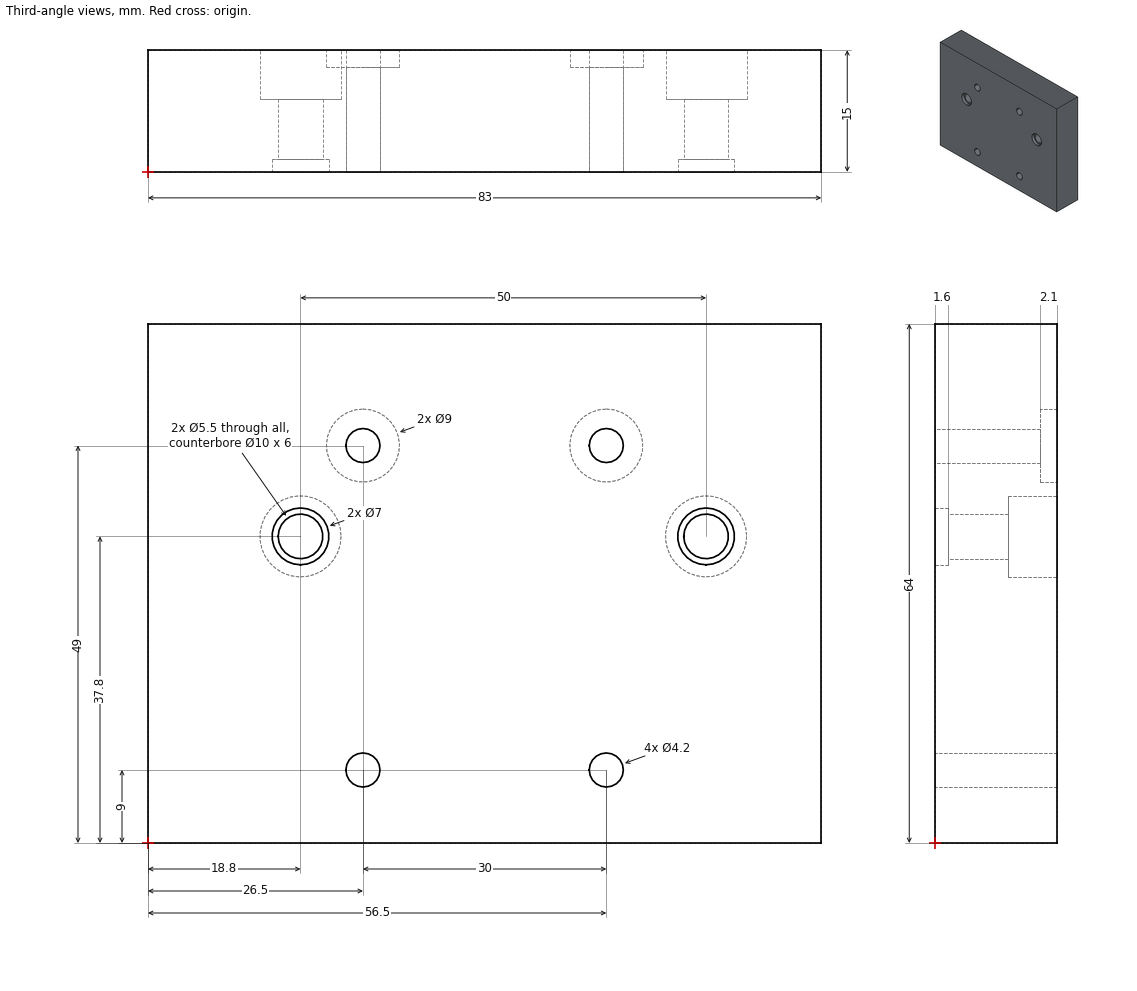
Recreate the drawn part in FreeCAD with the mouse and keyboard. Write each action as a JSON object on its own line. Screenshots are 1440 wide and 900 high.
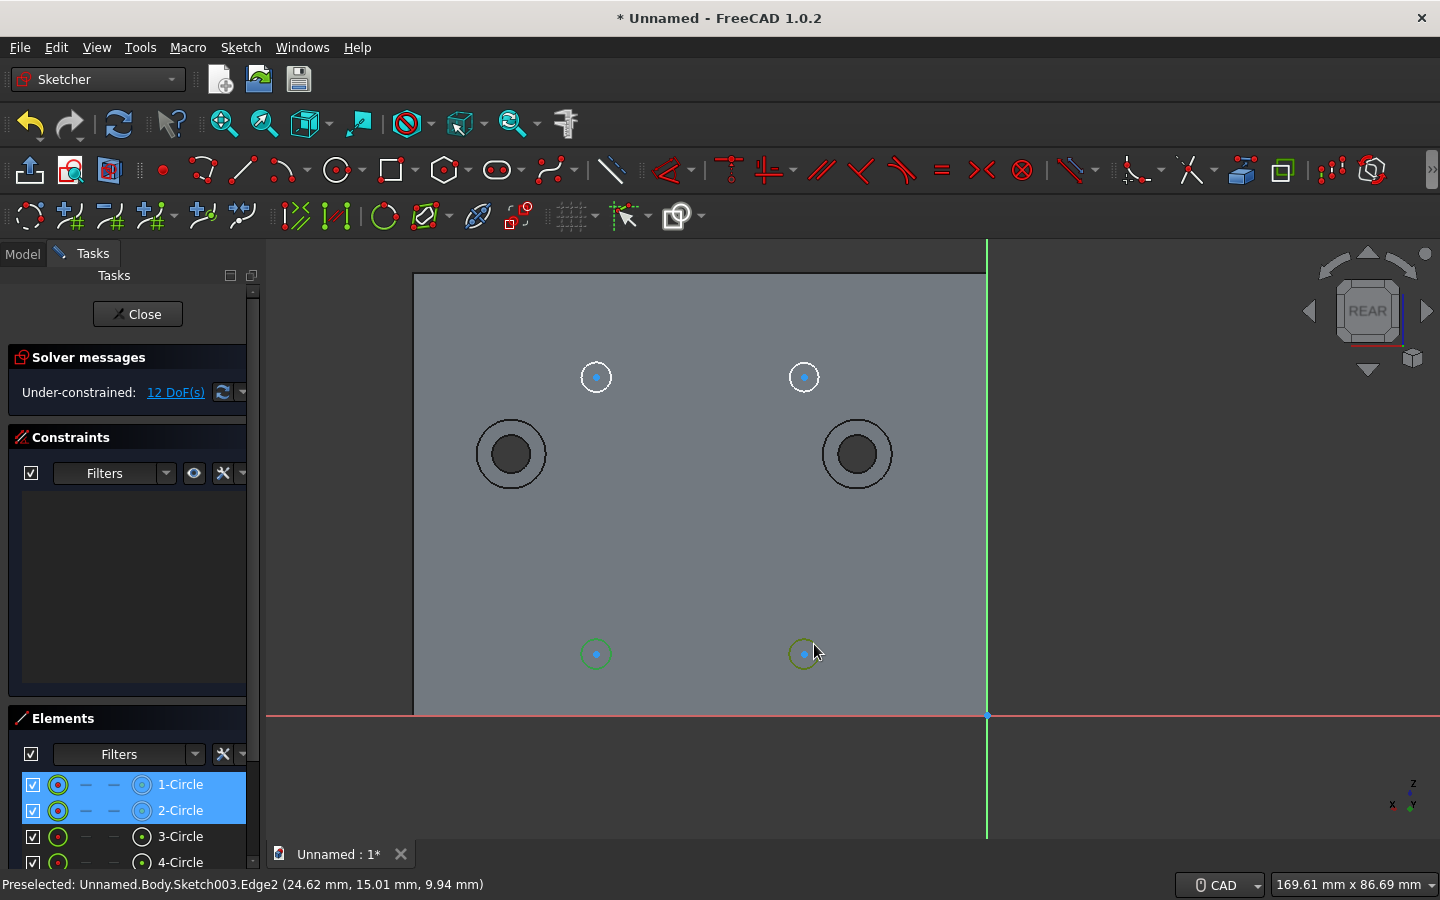
{"action": "left_click", "coordinate": [814, 367]}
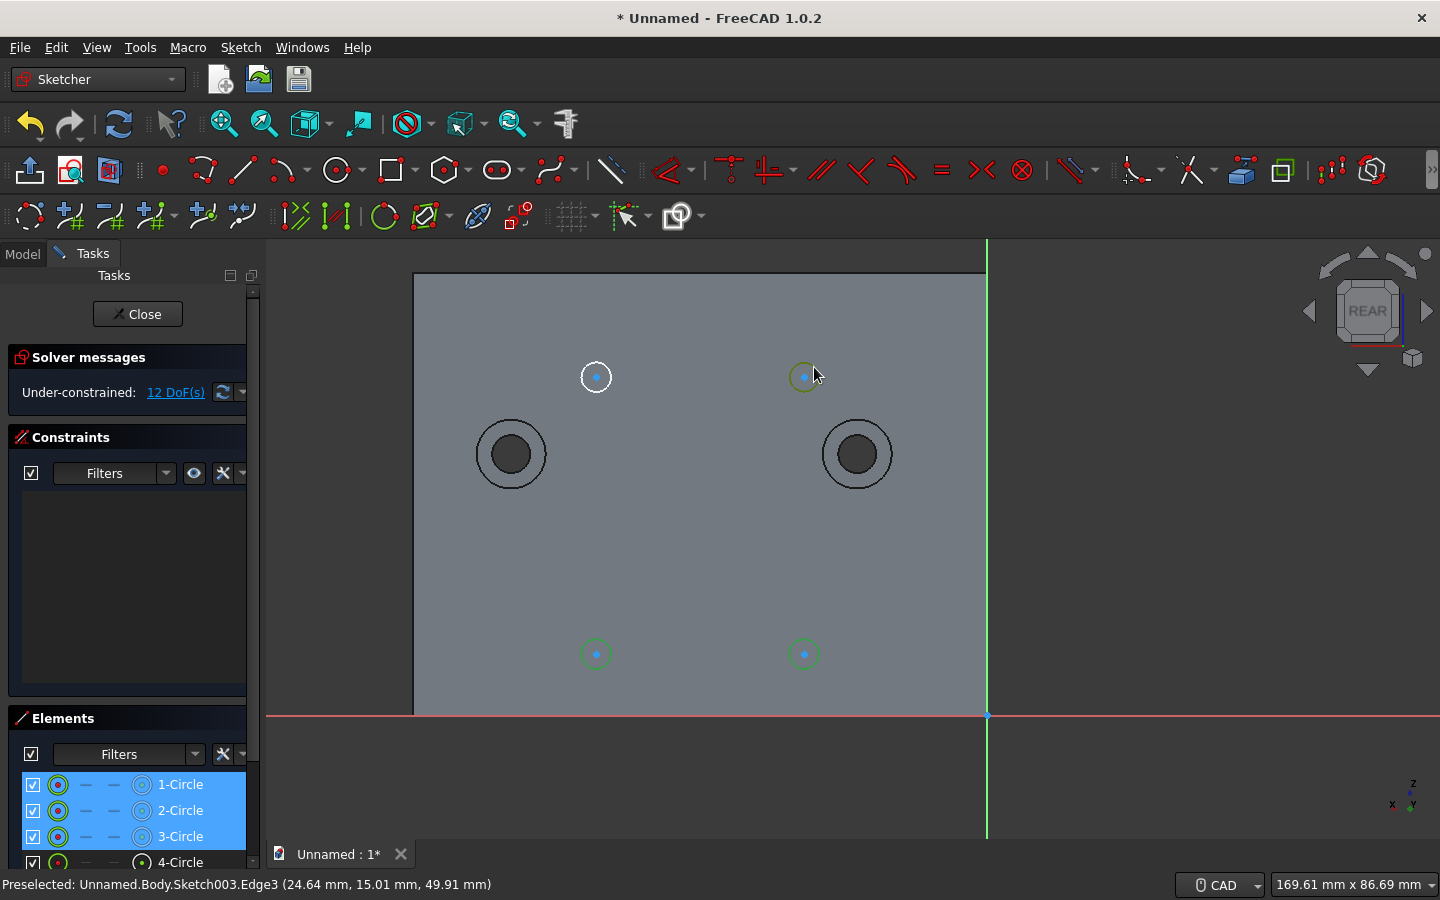
{"action": "left_click", "coordinate": [607, 367]}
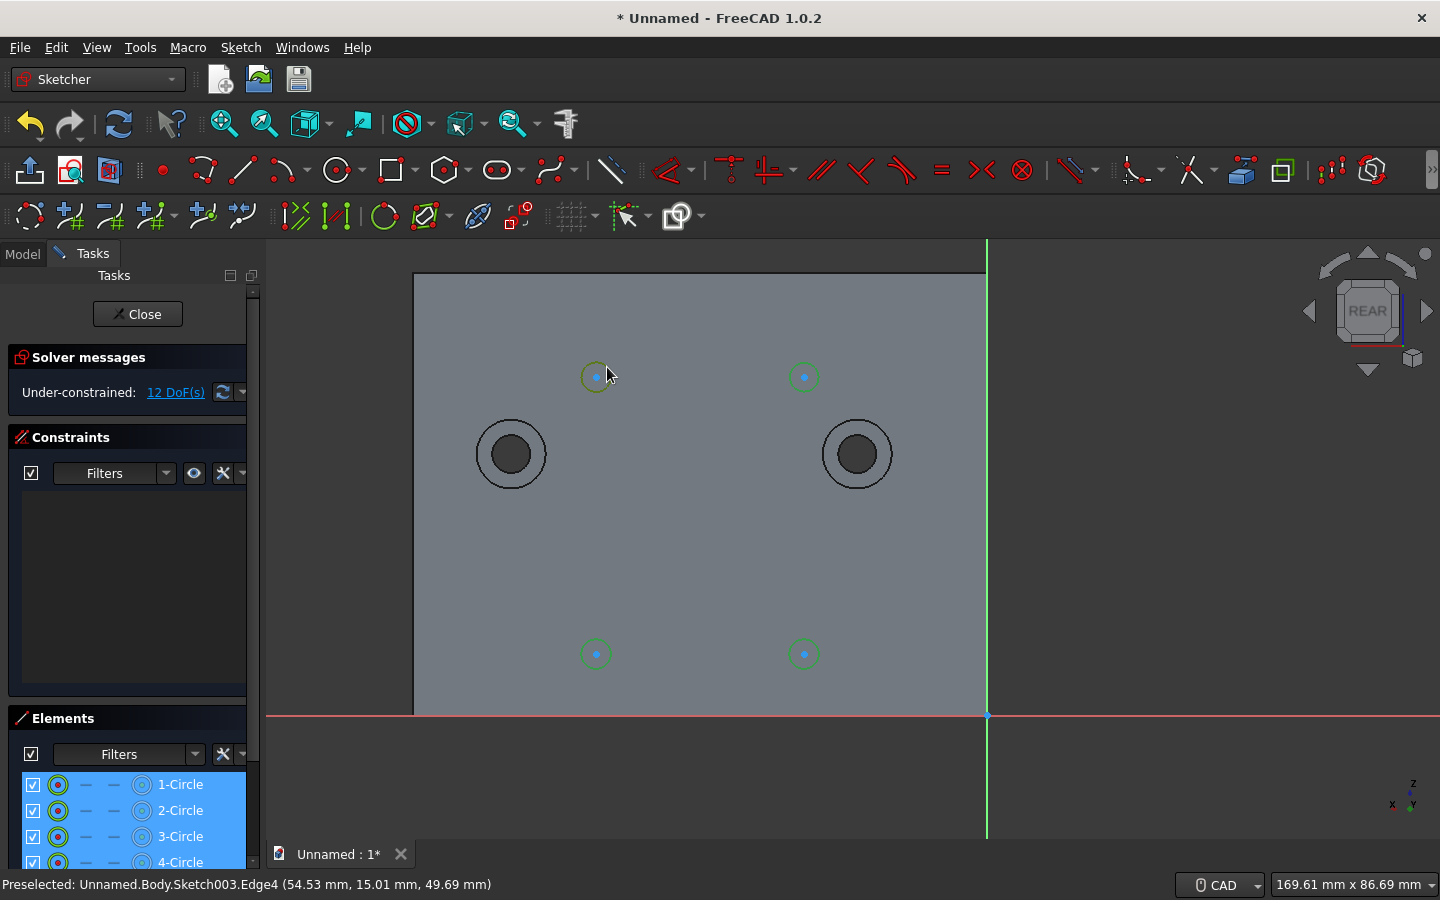
{"action": "left_click", "coordinate": [942, 170]}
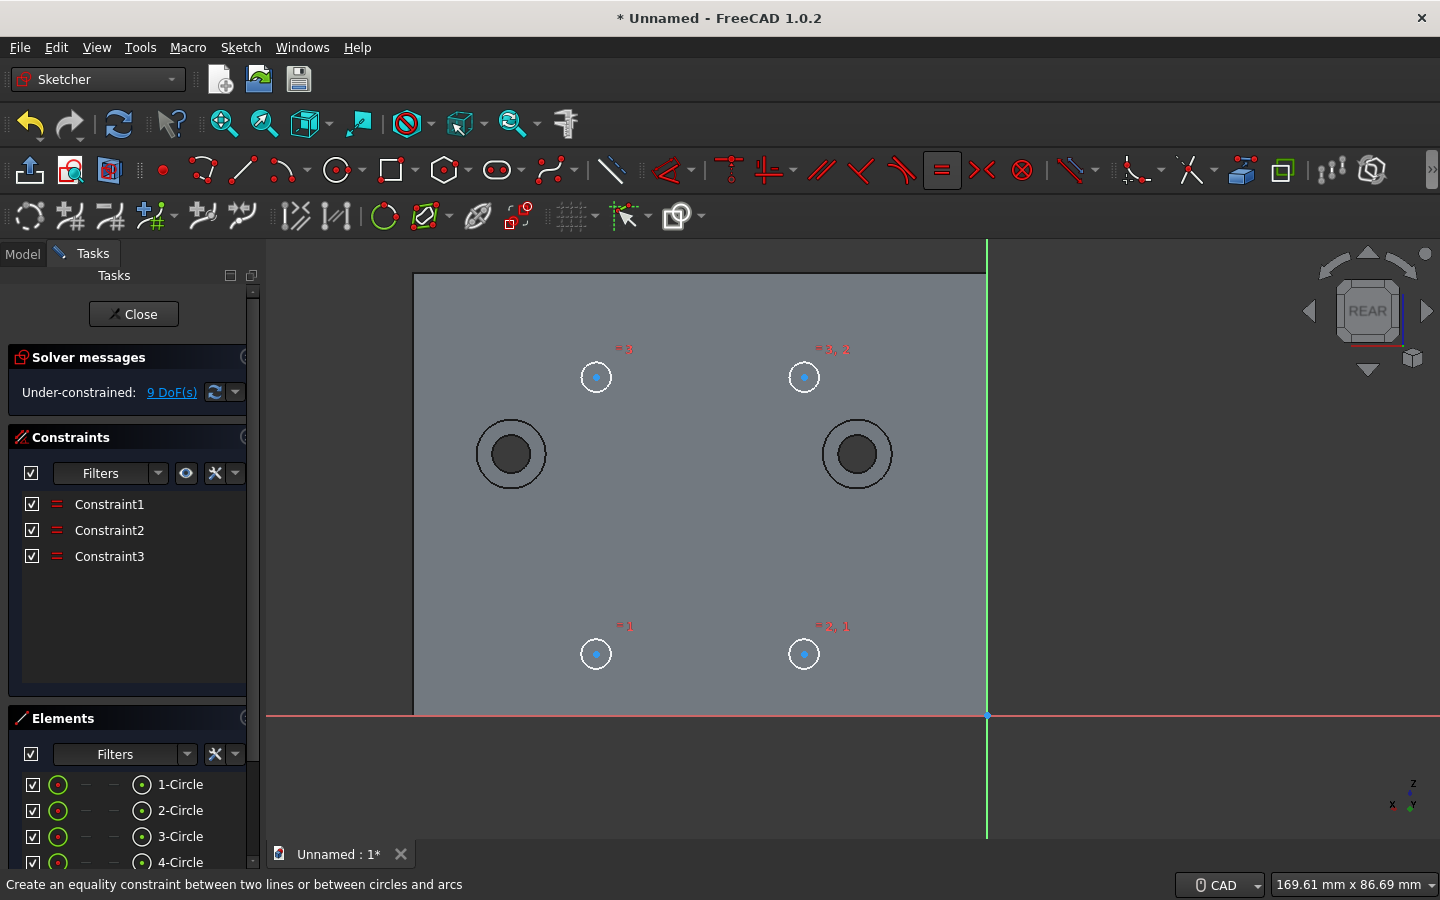
{"action": "left_click", "coordinate": [666, 170]}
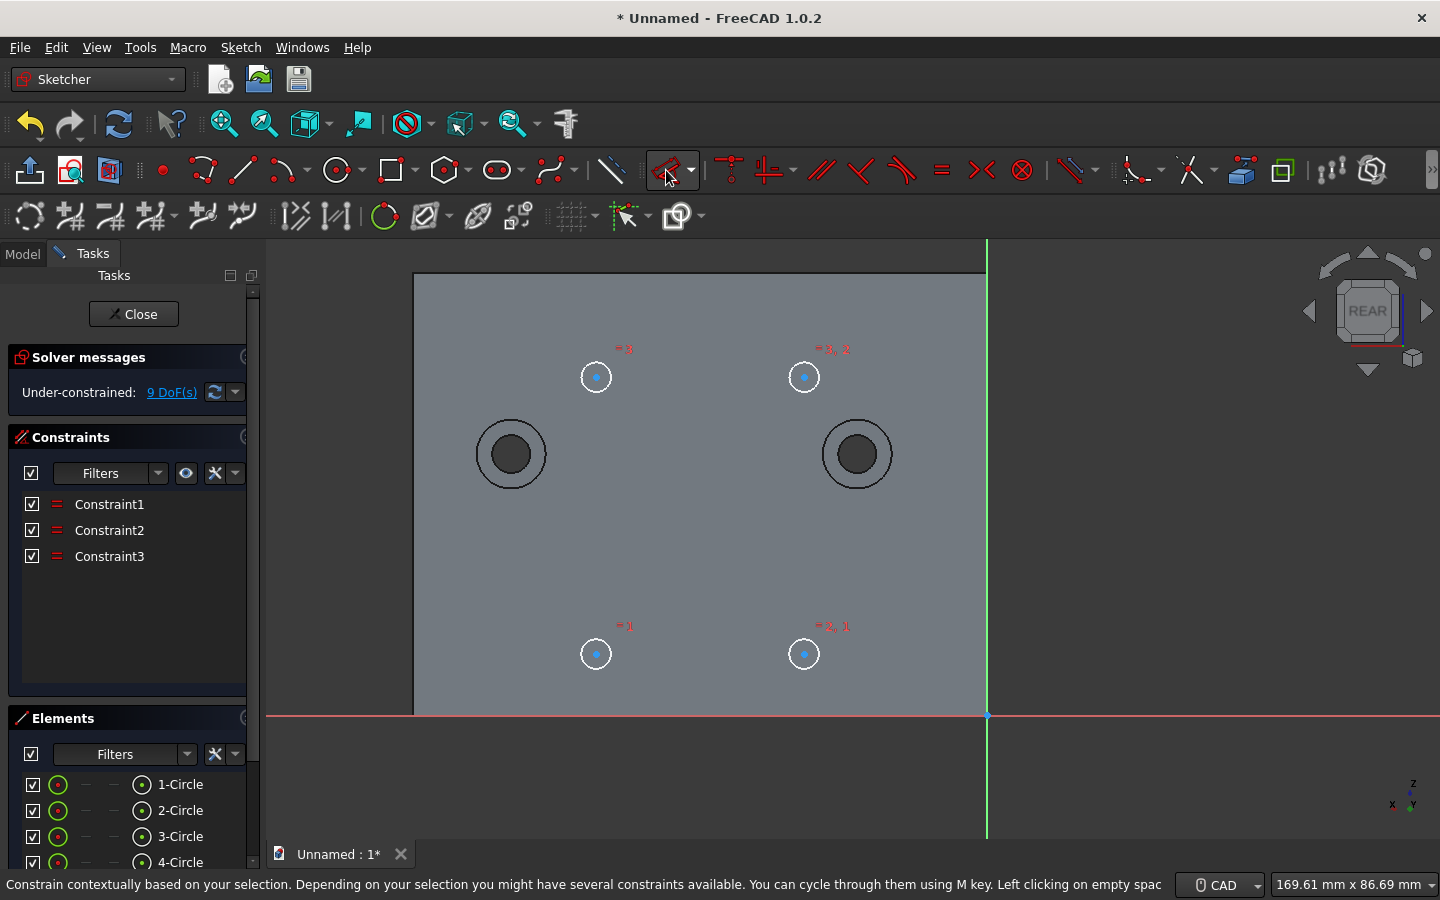
{"action": "scroll", "coordinate": [606, 644], "scroll_direction": "up", "scroll_amount": 2}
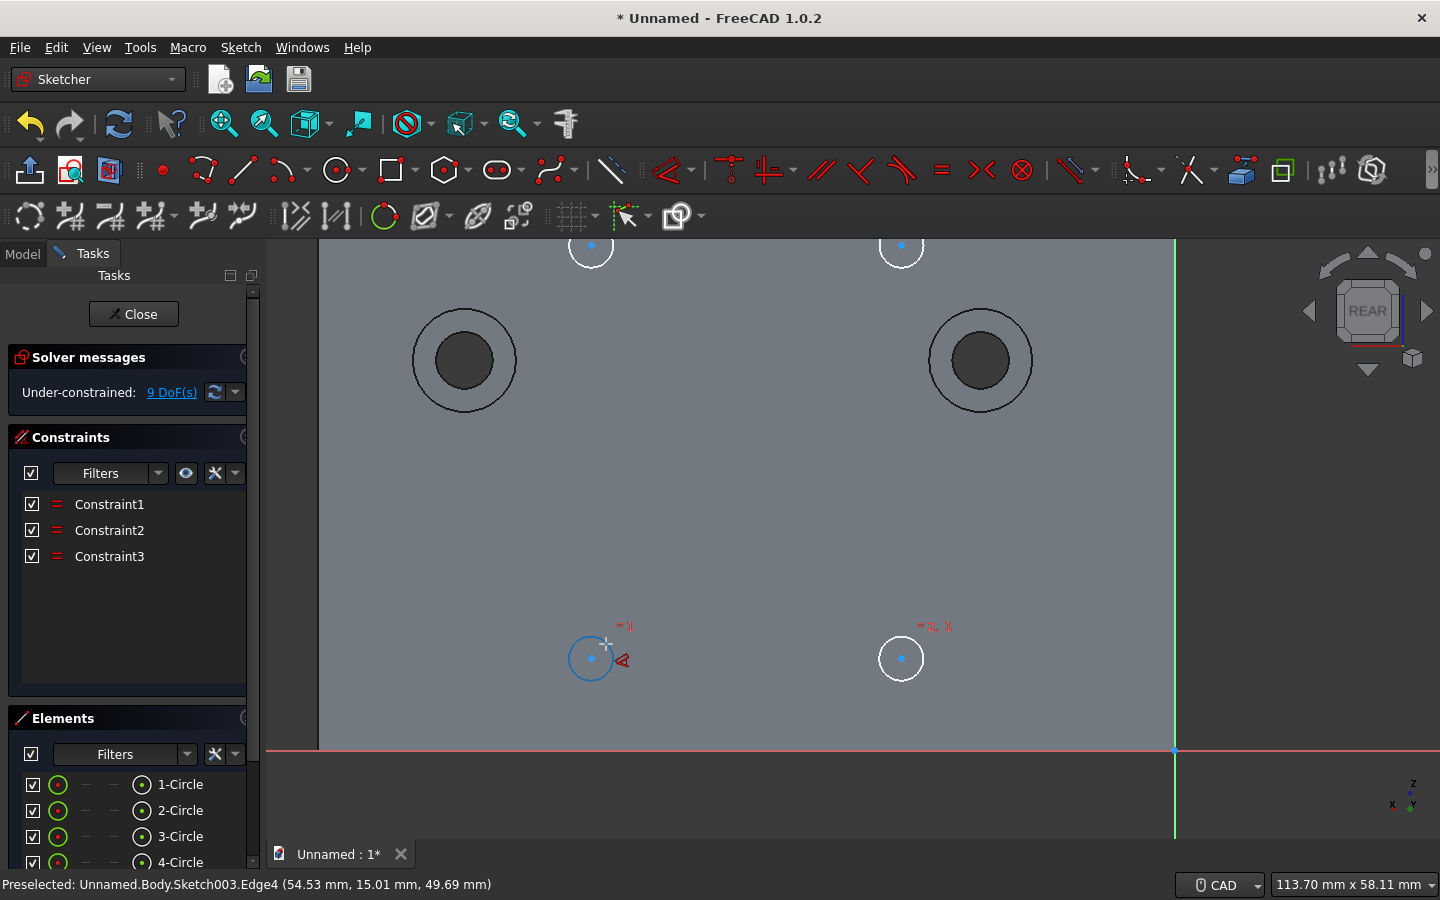
{"action": "left_click", "coordinate": [607, 643]}
{"action": "left_click", "coordinate": [630, 621]}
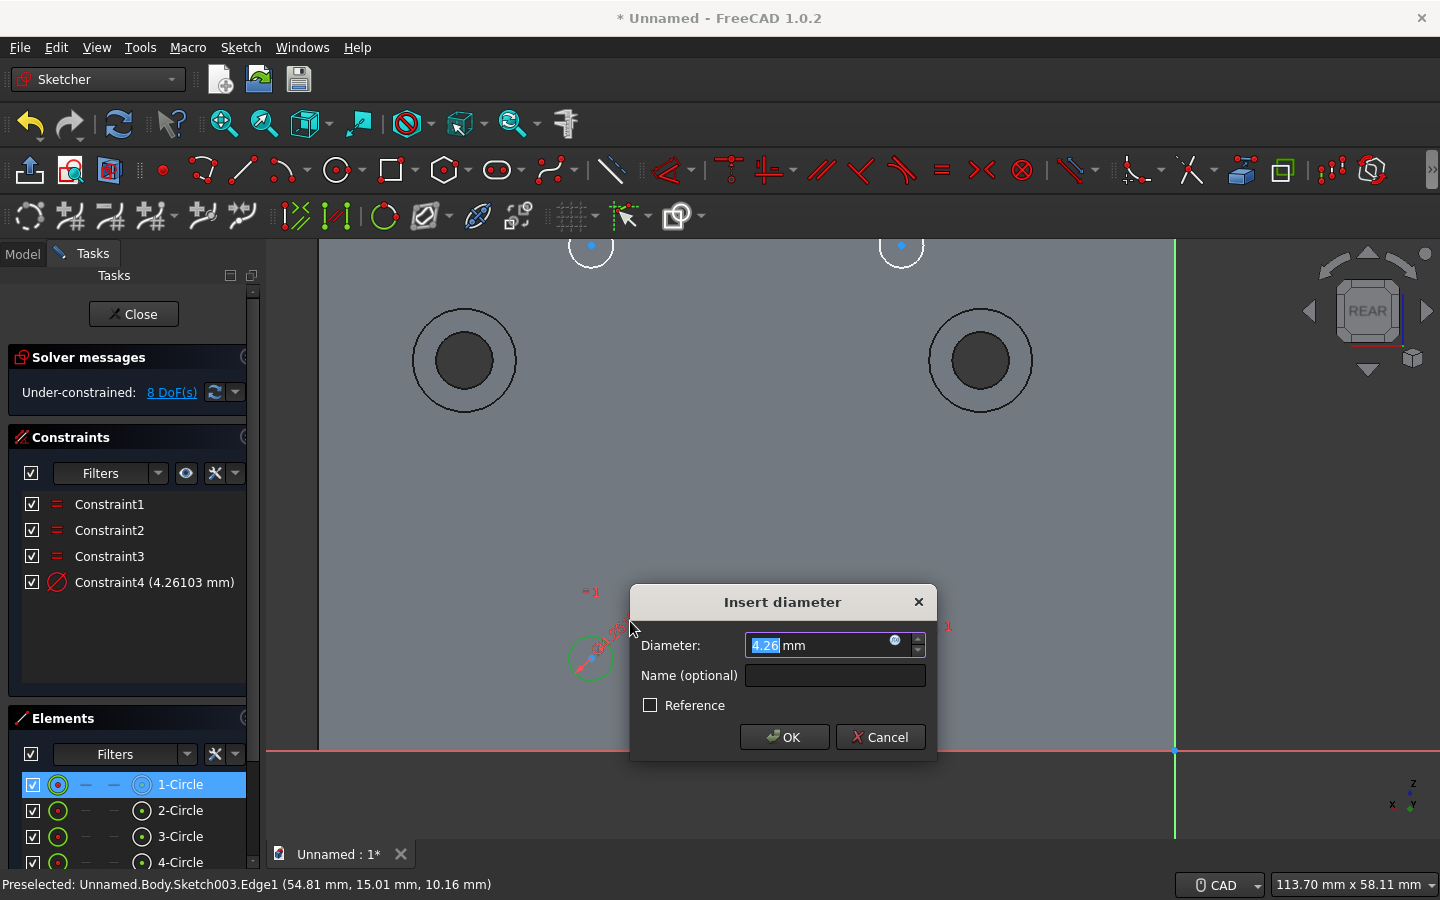
{"action": "type", "text": "4.2"}
{"action": "key", "text": "Return"}